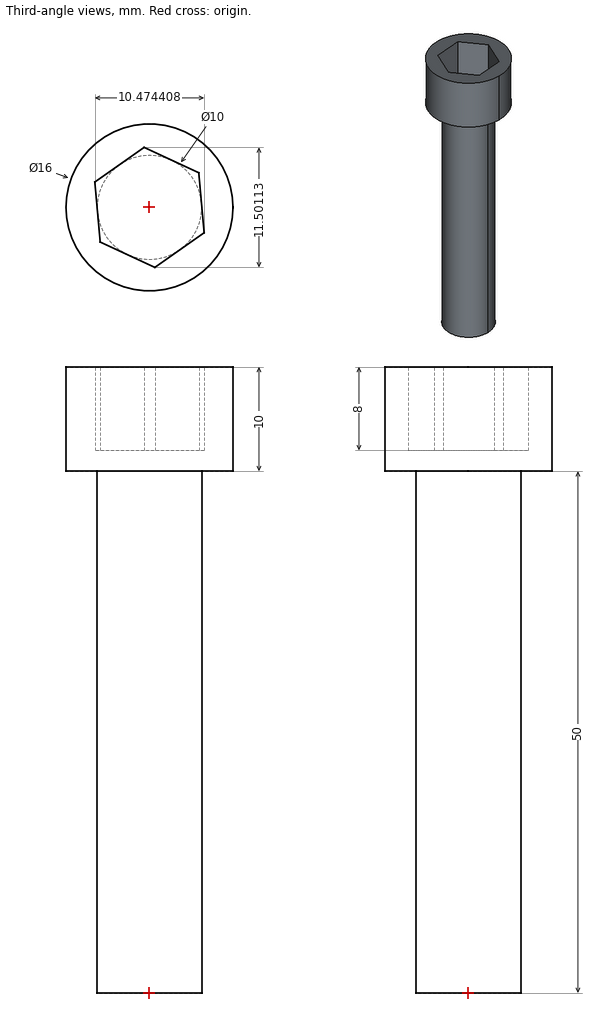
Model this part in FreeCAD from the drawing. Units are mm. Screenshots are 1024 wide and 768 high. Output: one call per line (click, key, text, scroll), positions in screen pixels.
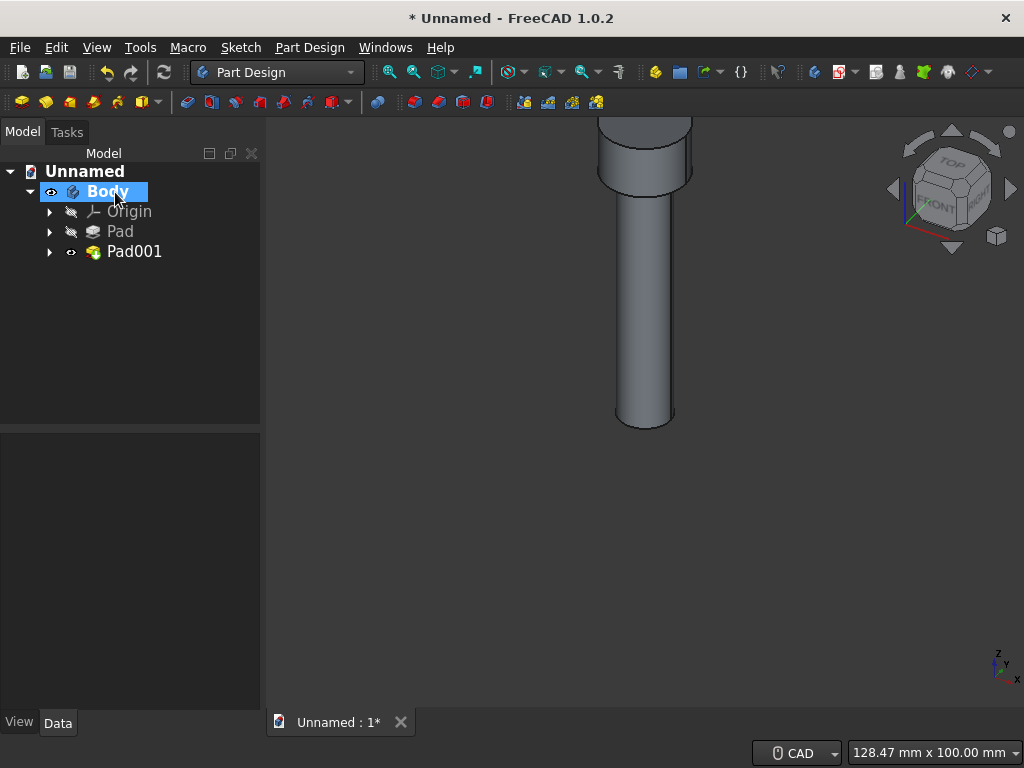
key(v)
key(f)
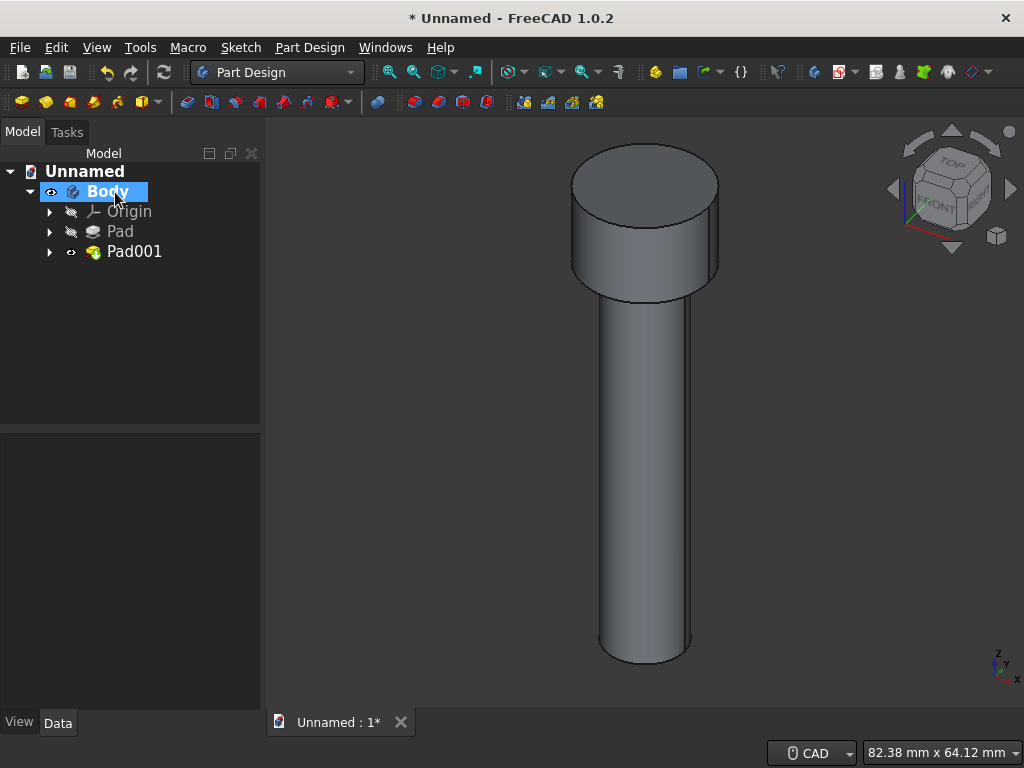
click(645, 185)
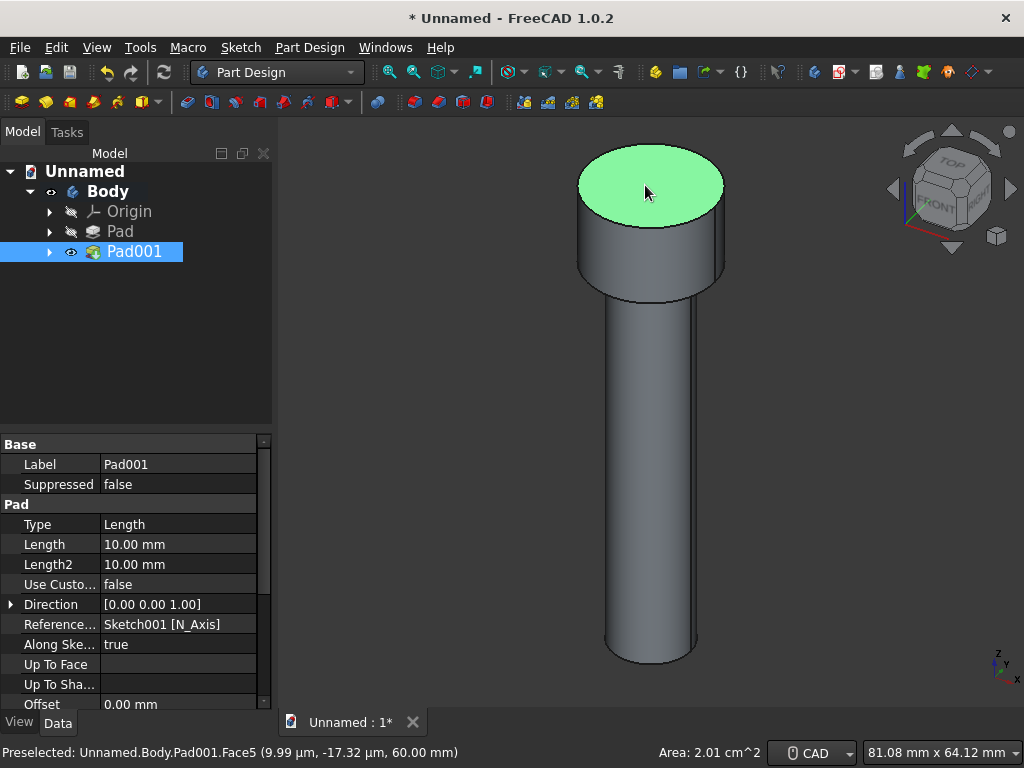
click(840, 72)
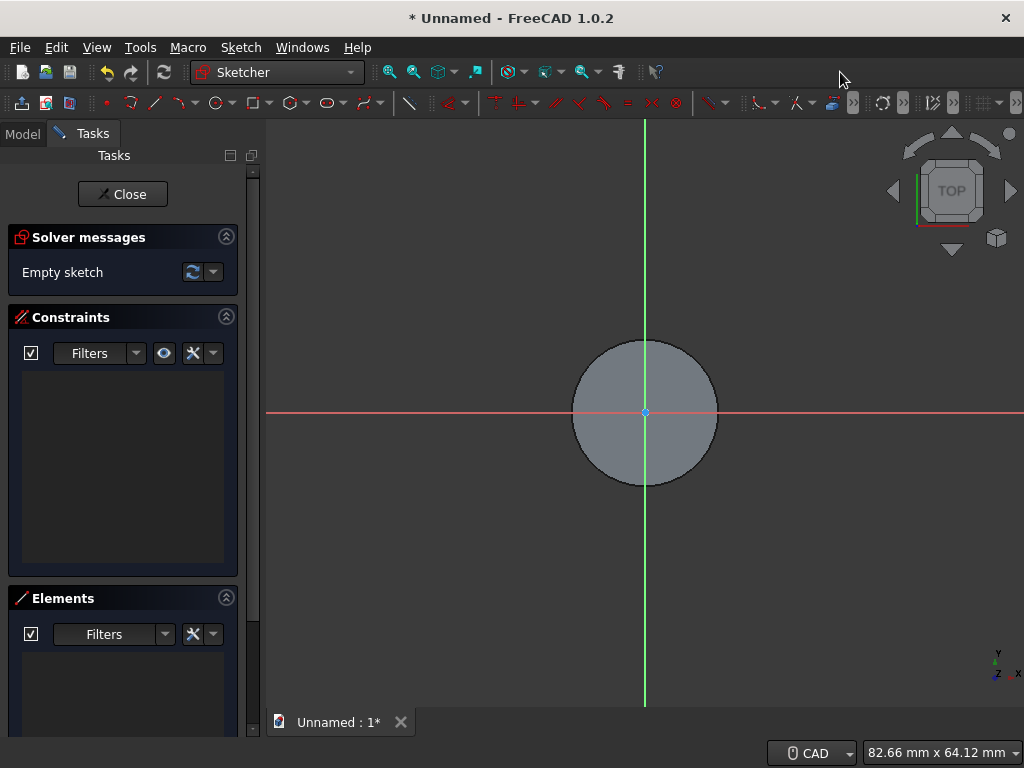
scroll(675, 413, up, 6)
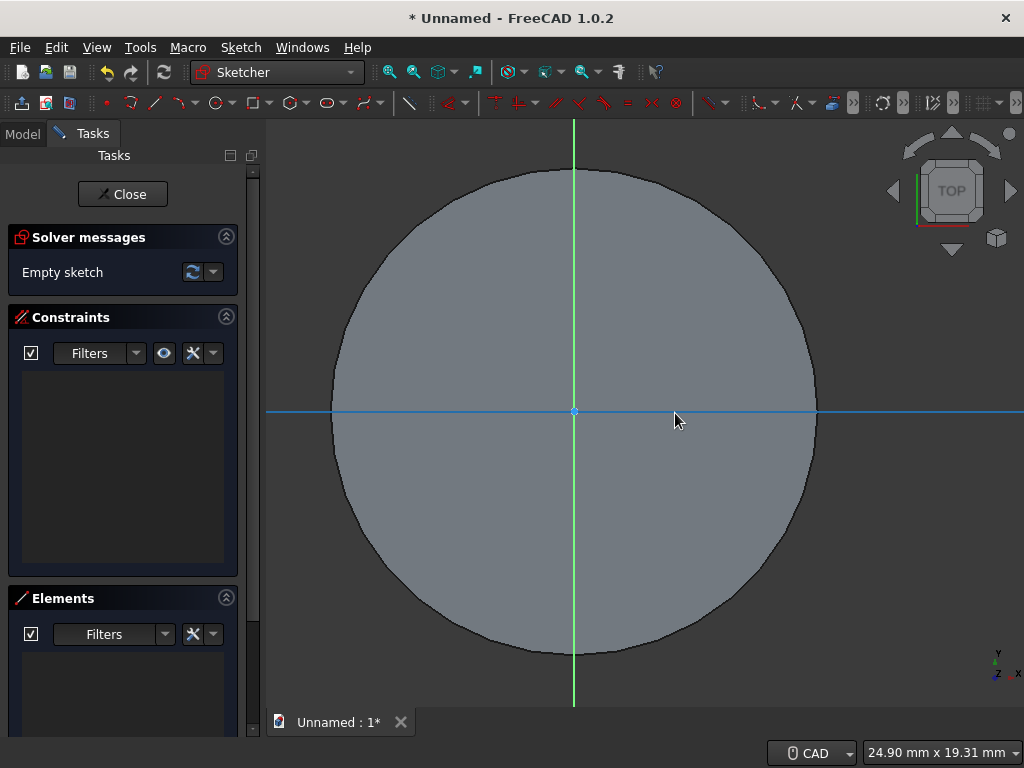
key(g)
key(p)
key(6)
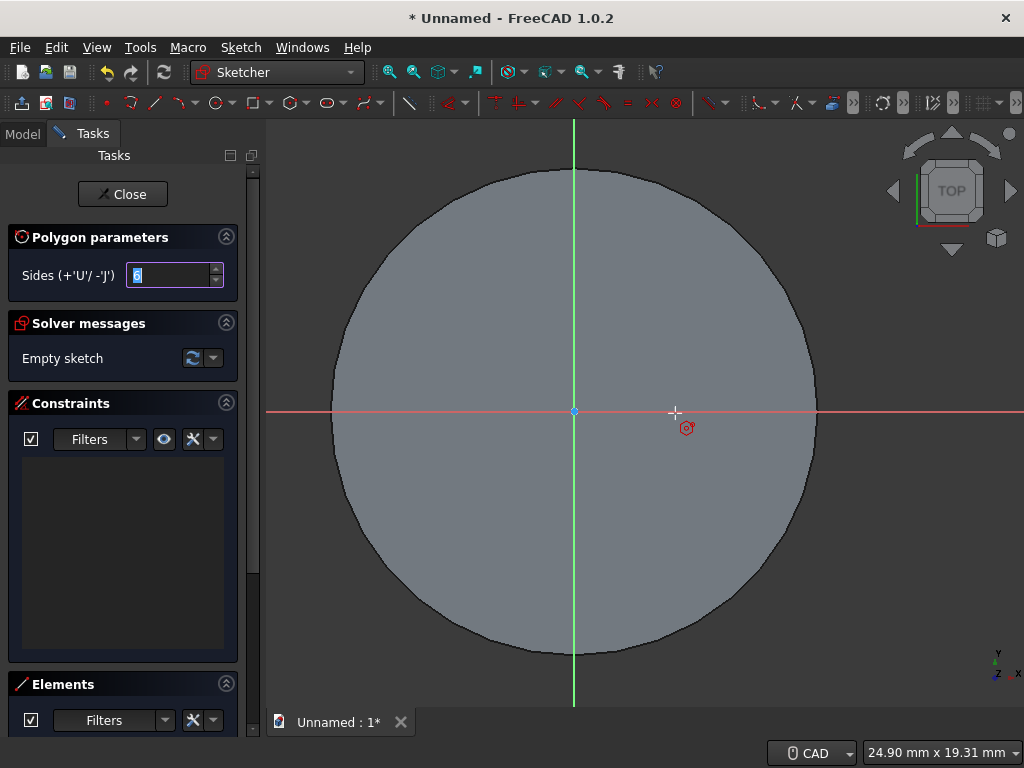
click(574, 412)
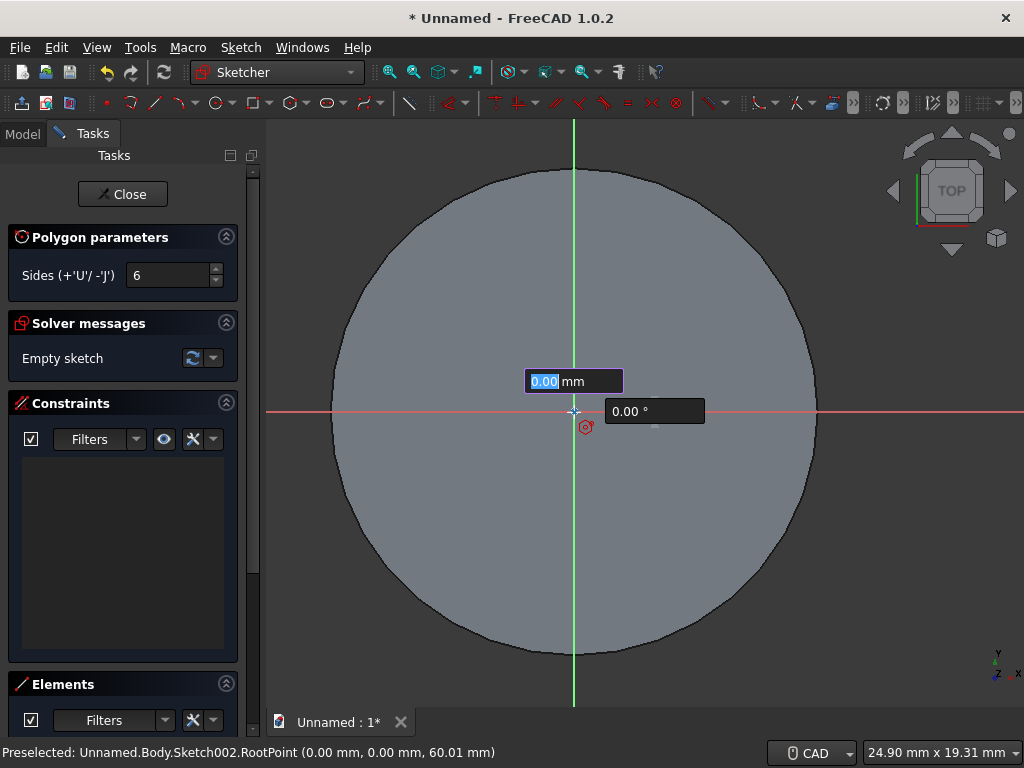
click(718, 311)
right_click(718, 311)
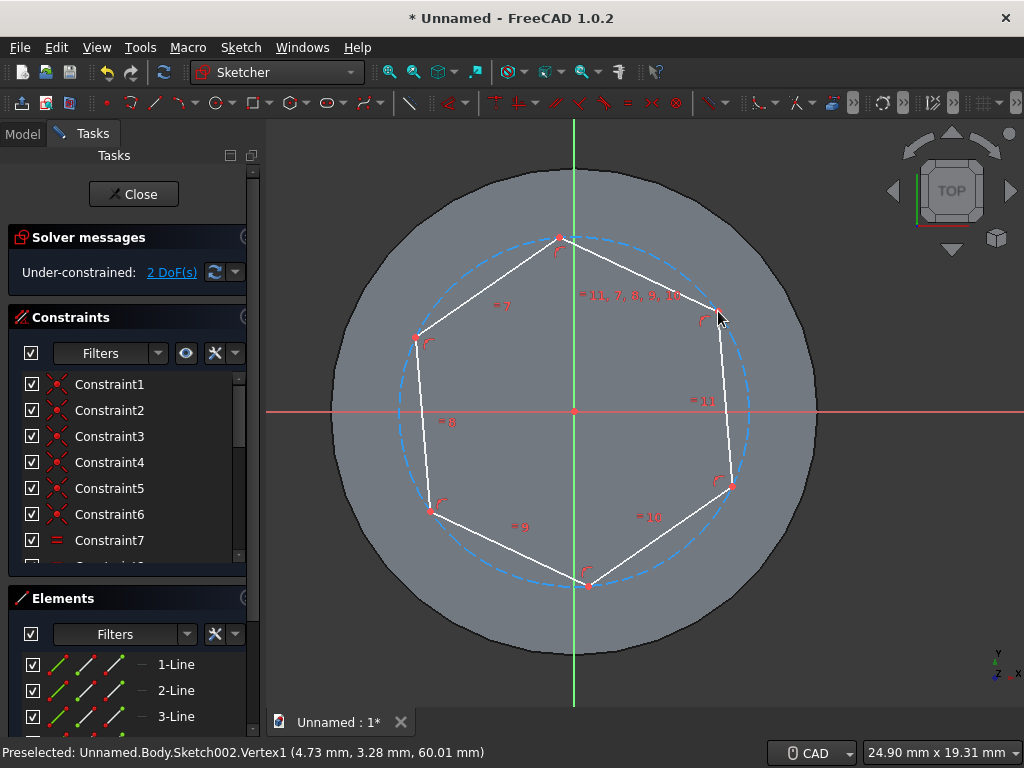
click(416, 337)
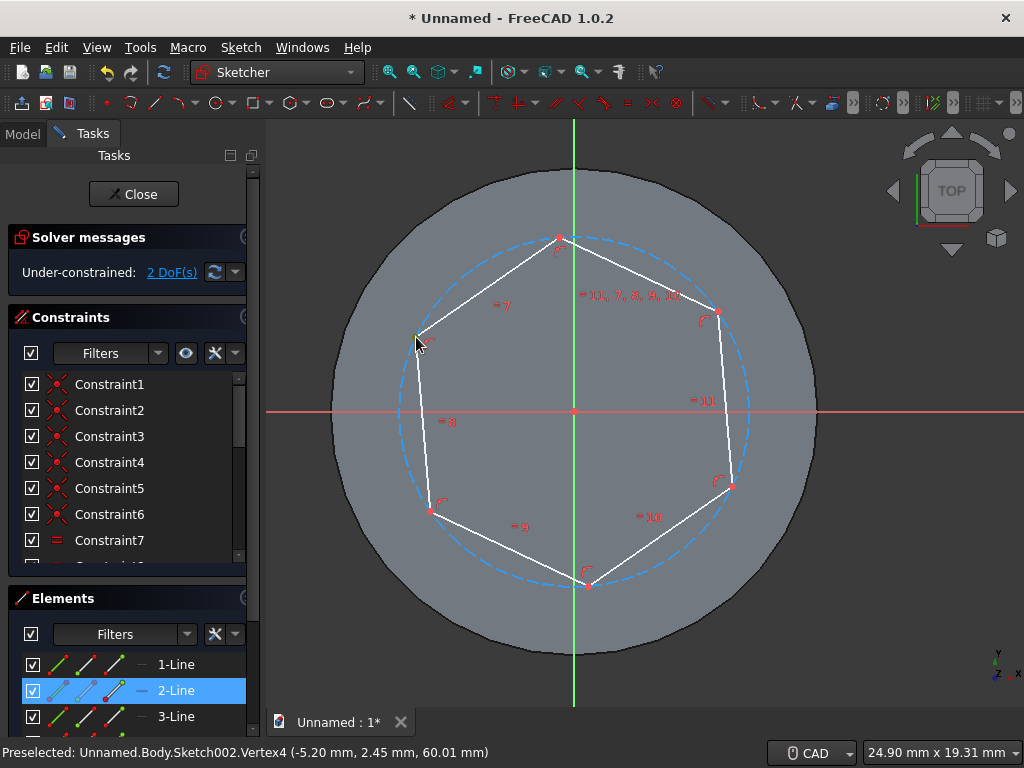
click(733, 487)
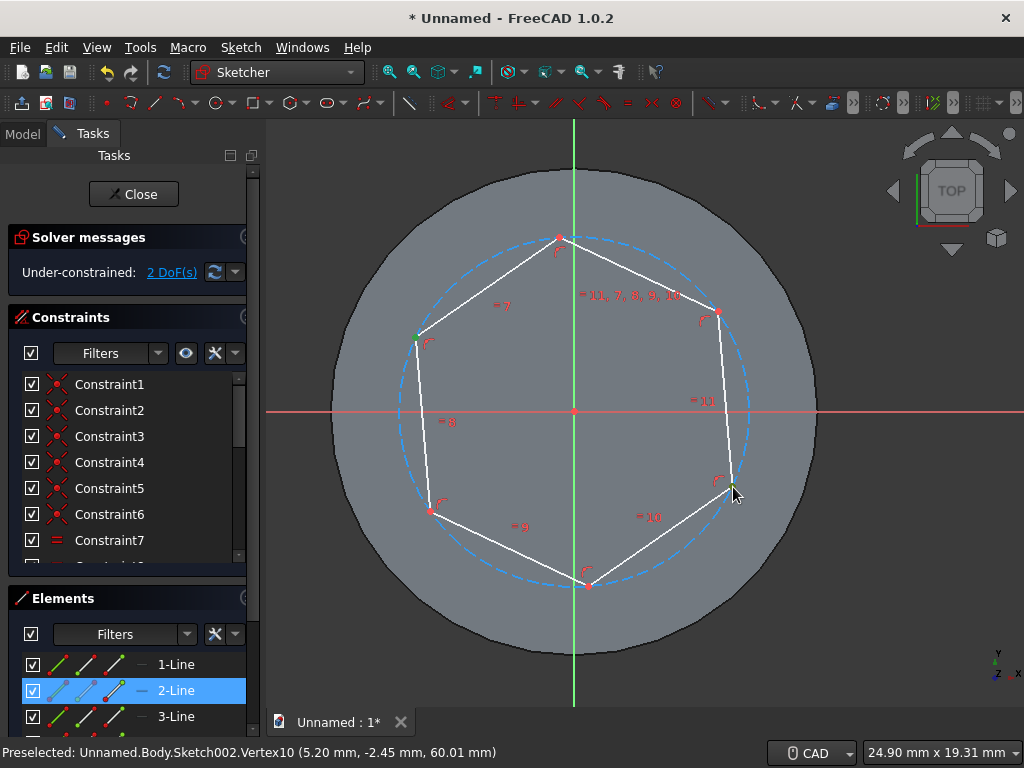
key(l)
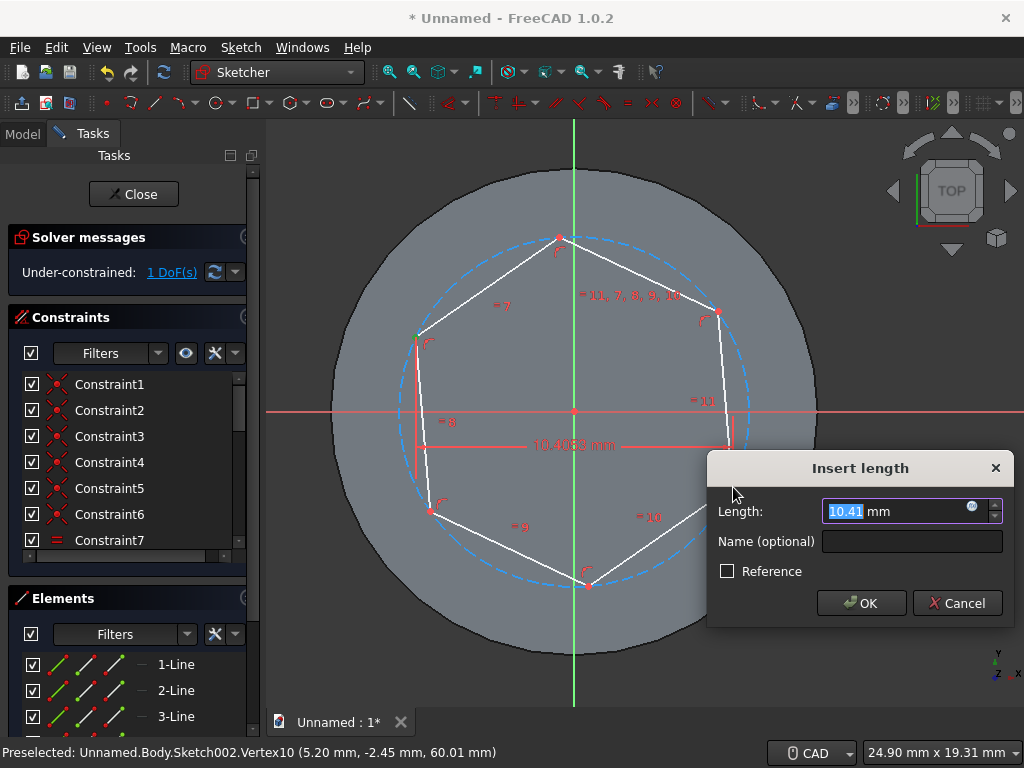
text(10.474408)
key(Return)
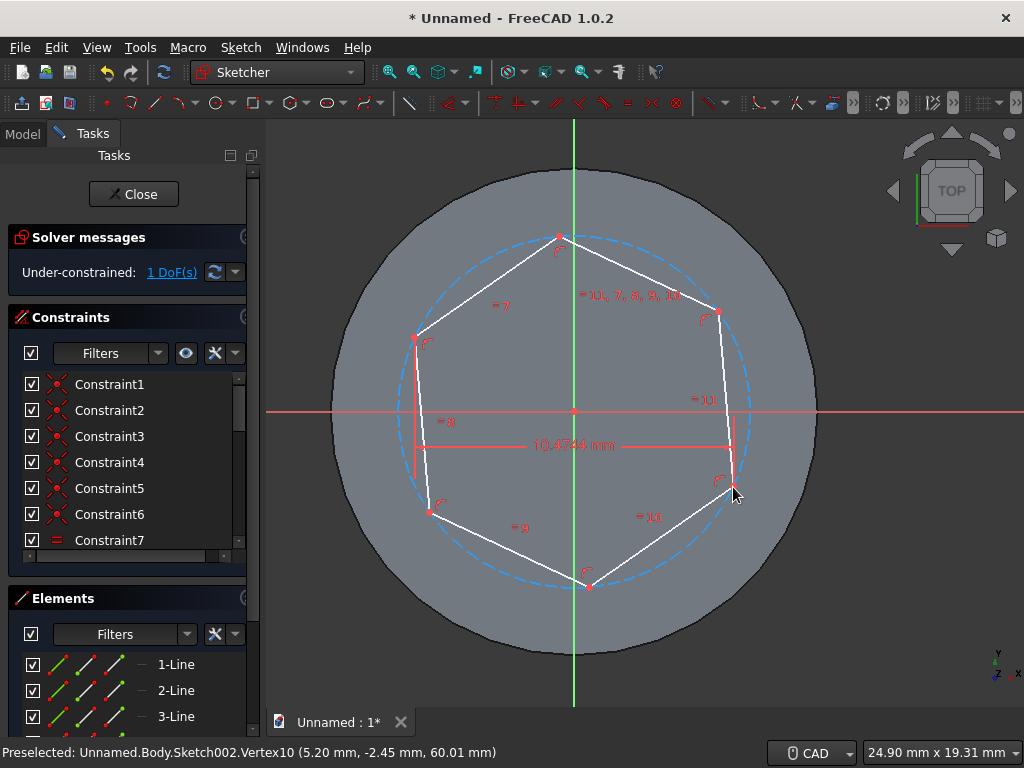
click(589, 587)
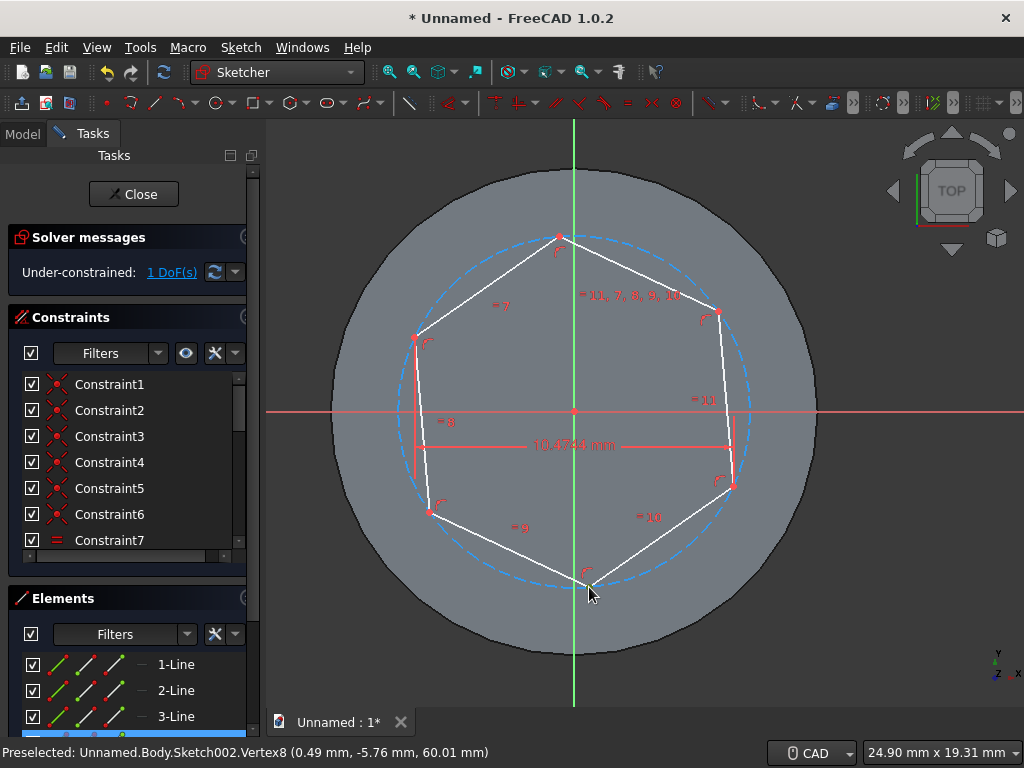
click(559, 236)